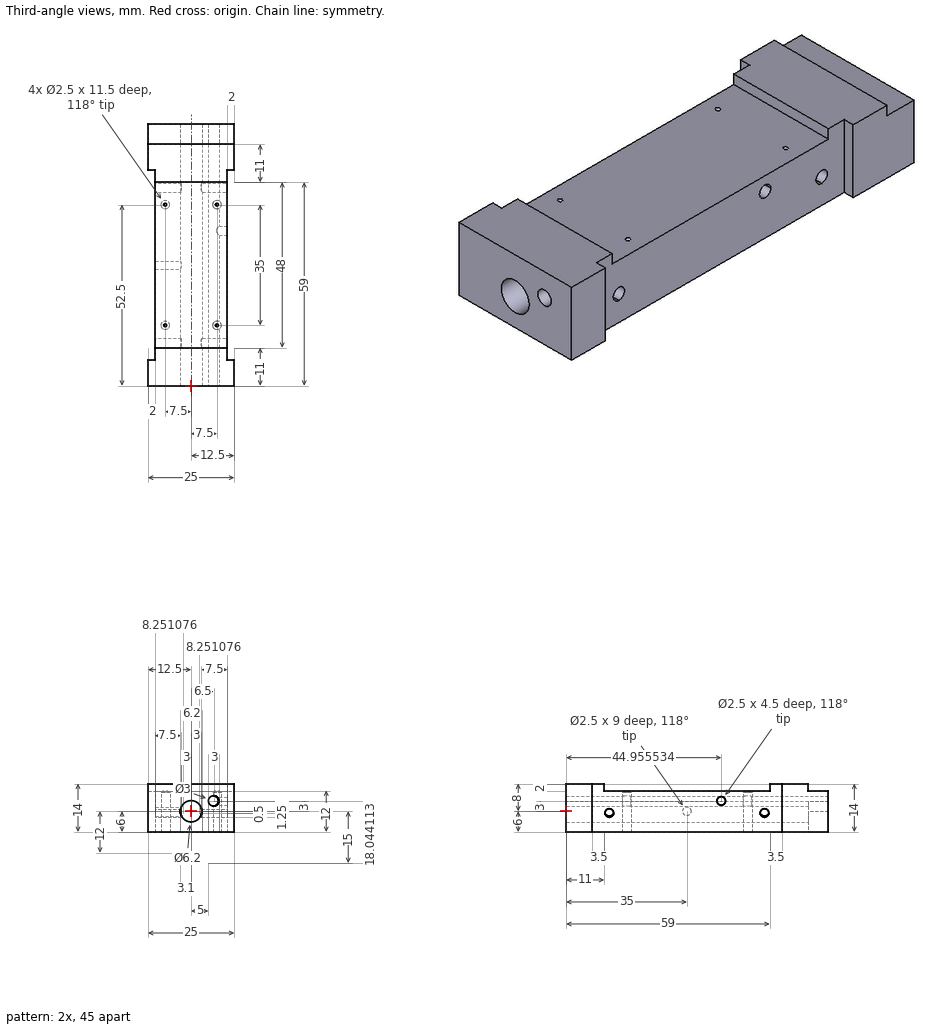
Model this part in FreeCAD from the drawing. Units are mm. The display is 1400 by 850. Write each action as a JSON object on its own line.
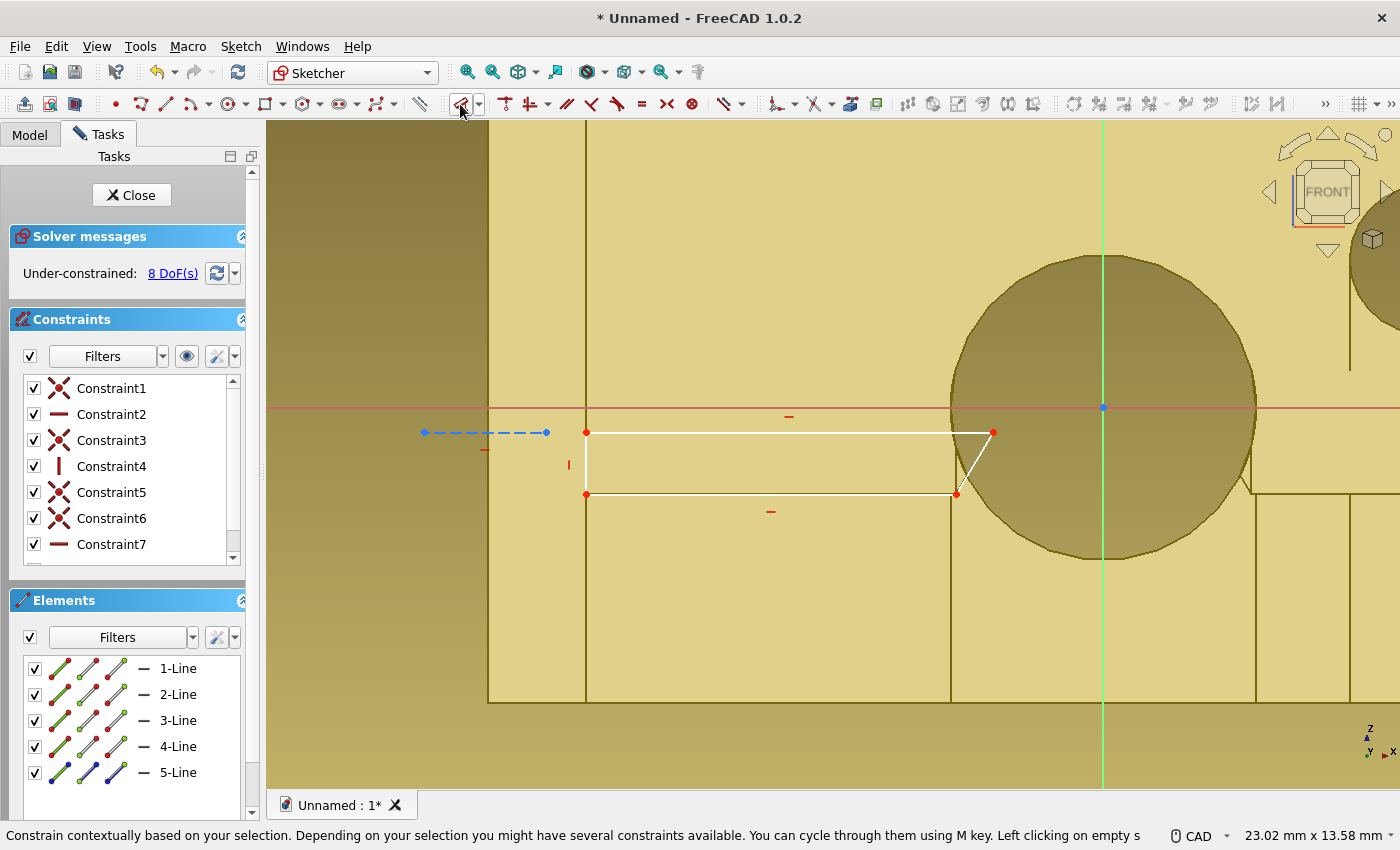
{"action": "left_click", "coordinate": [956, 495]}
{"action": "left_click", "coordinate": [1030, 529]}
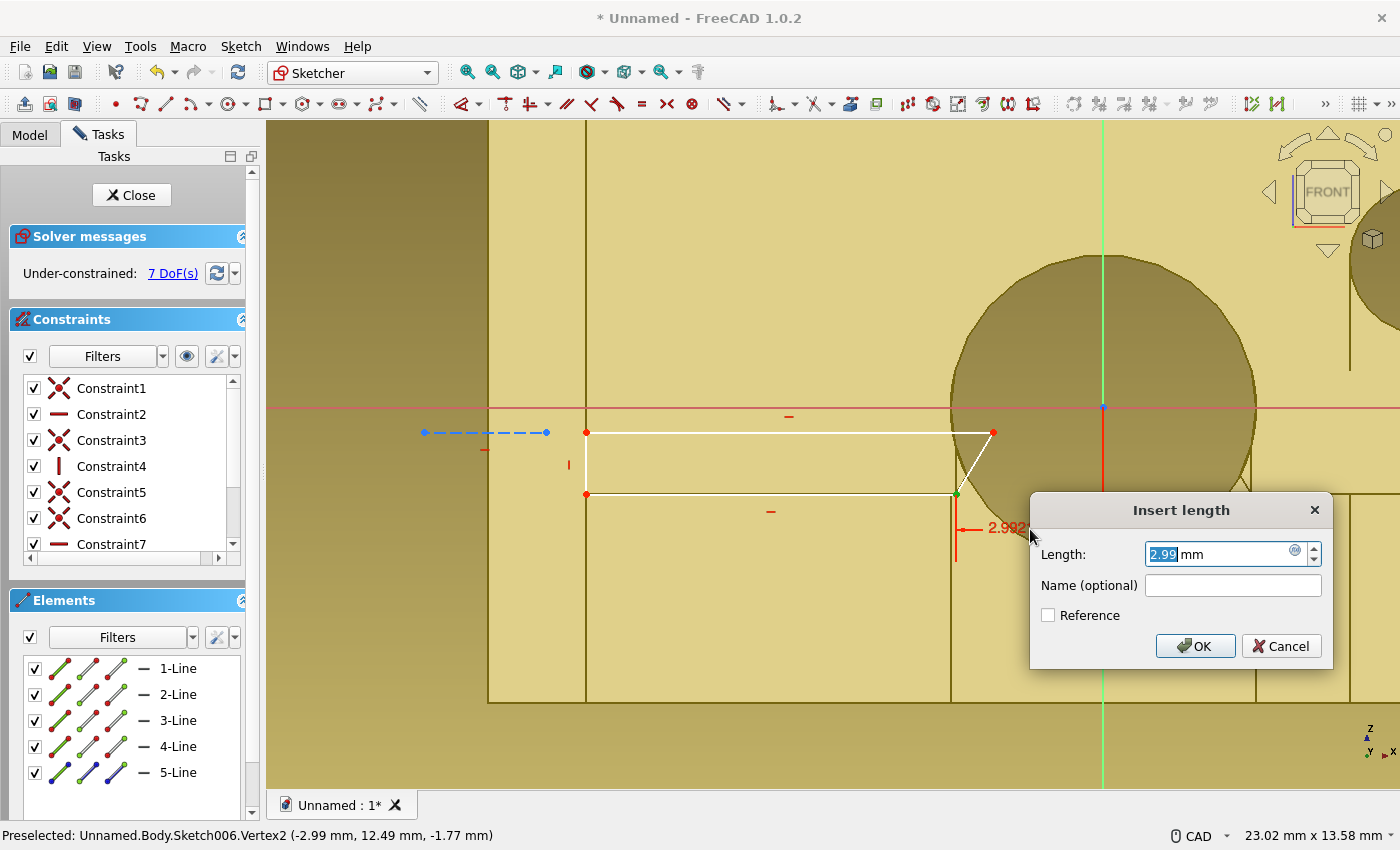
{"action": "type", "text": "3"}
{"action": "key", "text": "Return"}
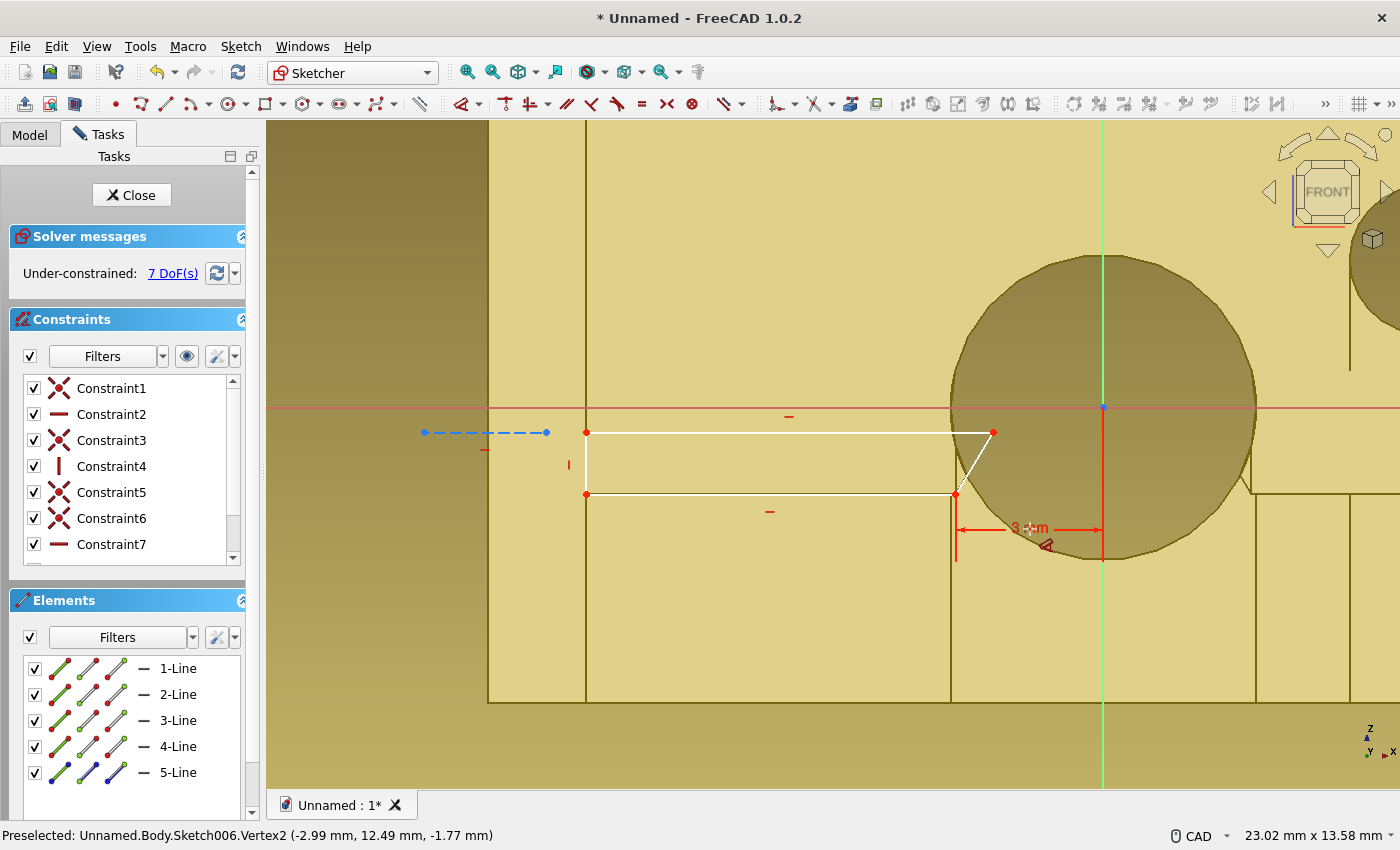
{"action": "left_click", "coordinate": [845, 495]}
{"action": "left_click", "coordinate": [771, 529]}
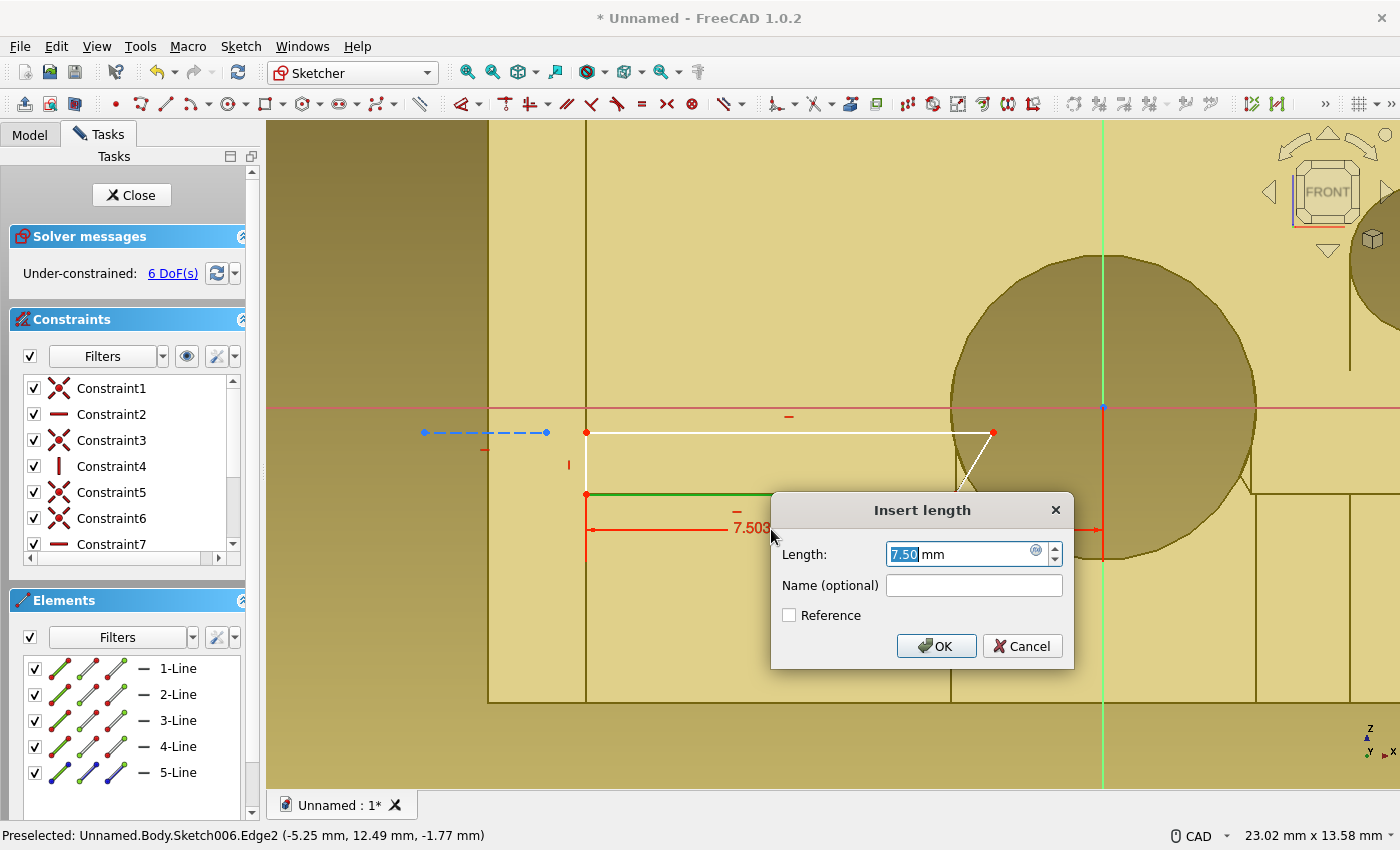
{"action": "type", "text": "7.5"}
{"action": "key", "text": "Return"}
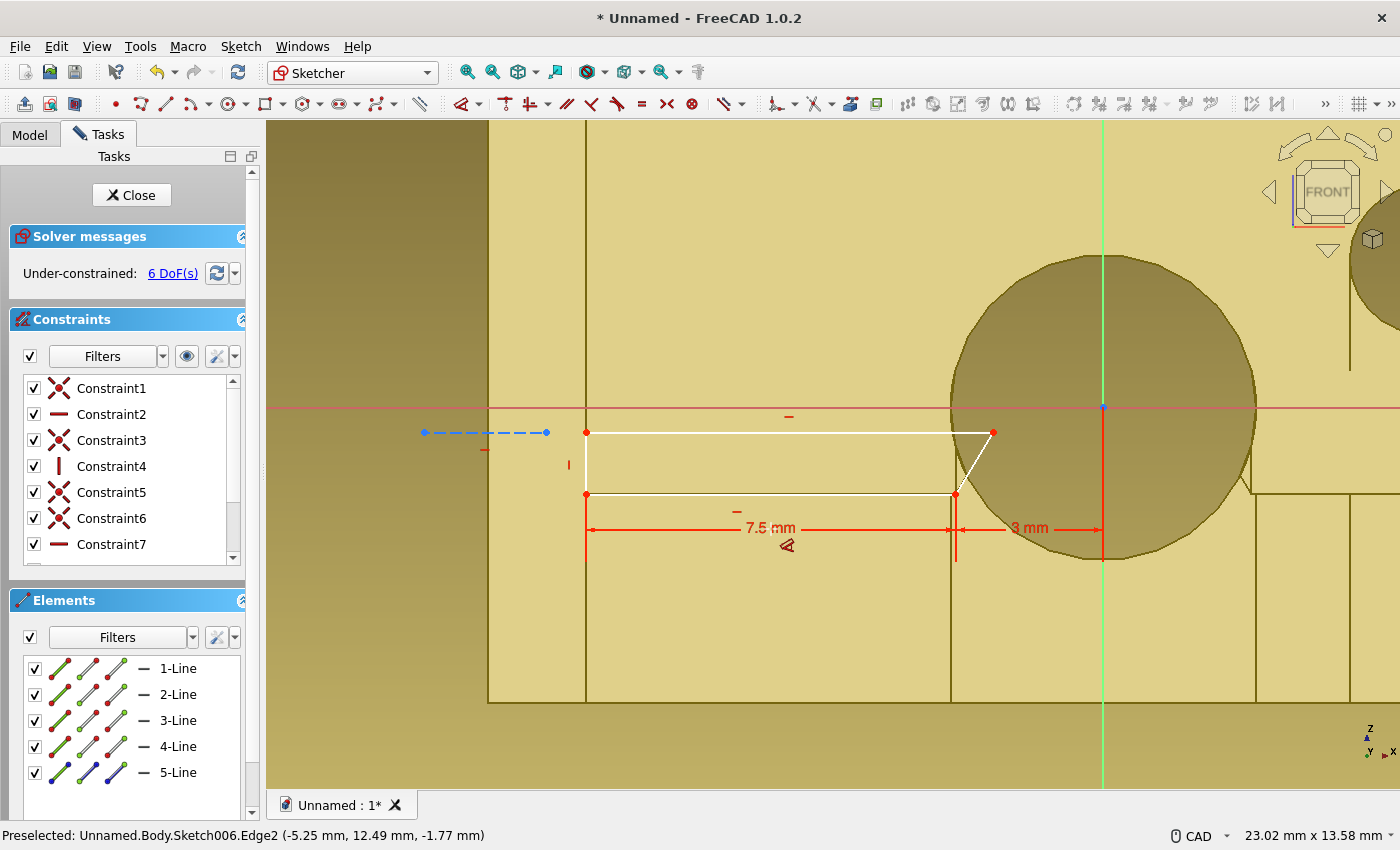
{"action": "left_click", "coordinate": [586, 476]}
{"action": "left_click", "coordinate": [552, 464]}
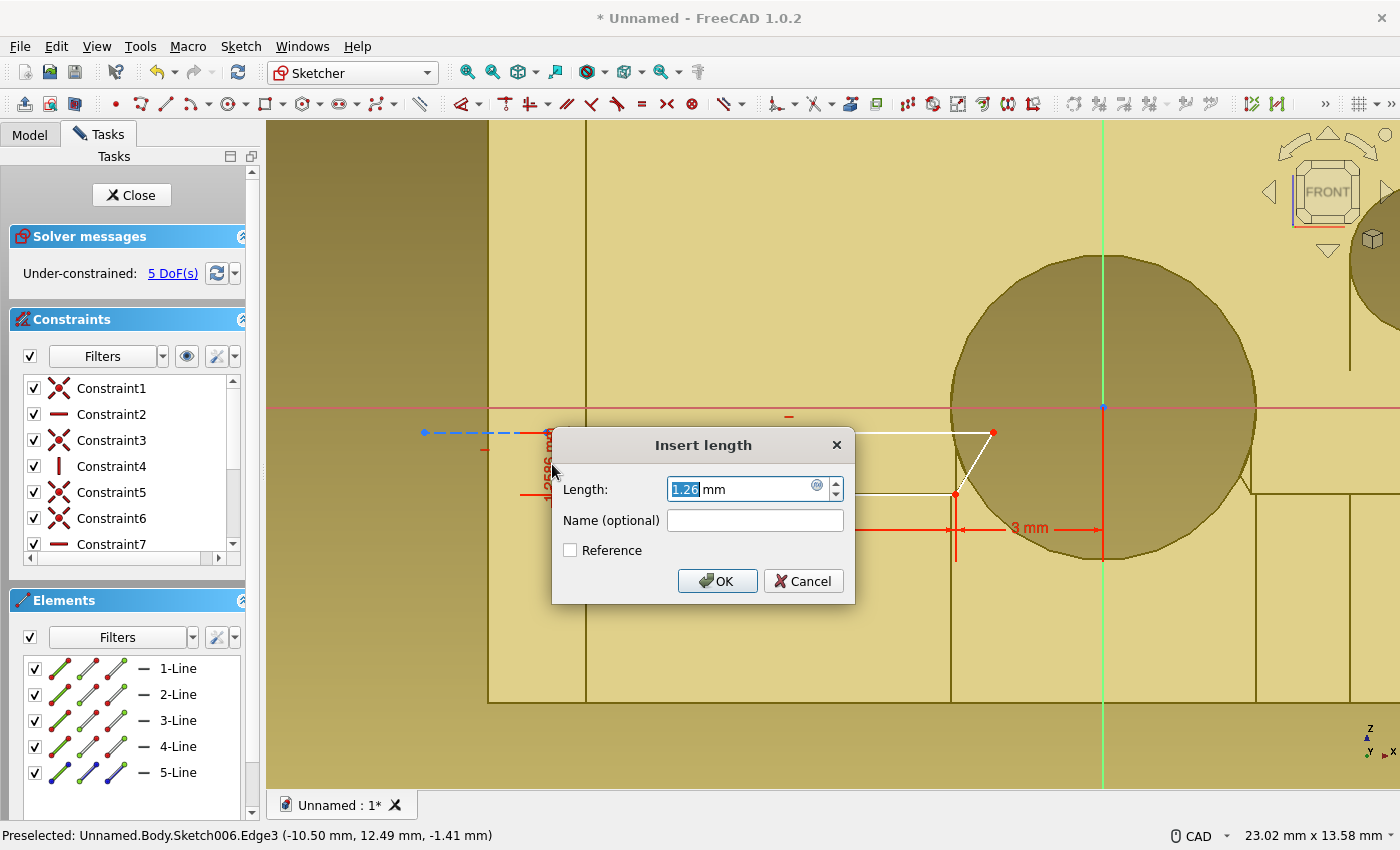
{"action": "type", "text": "1.25"}
{"action": "key", "text": "Return"}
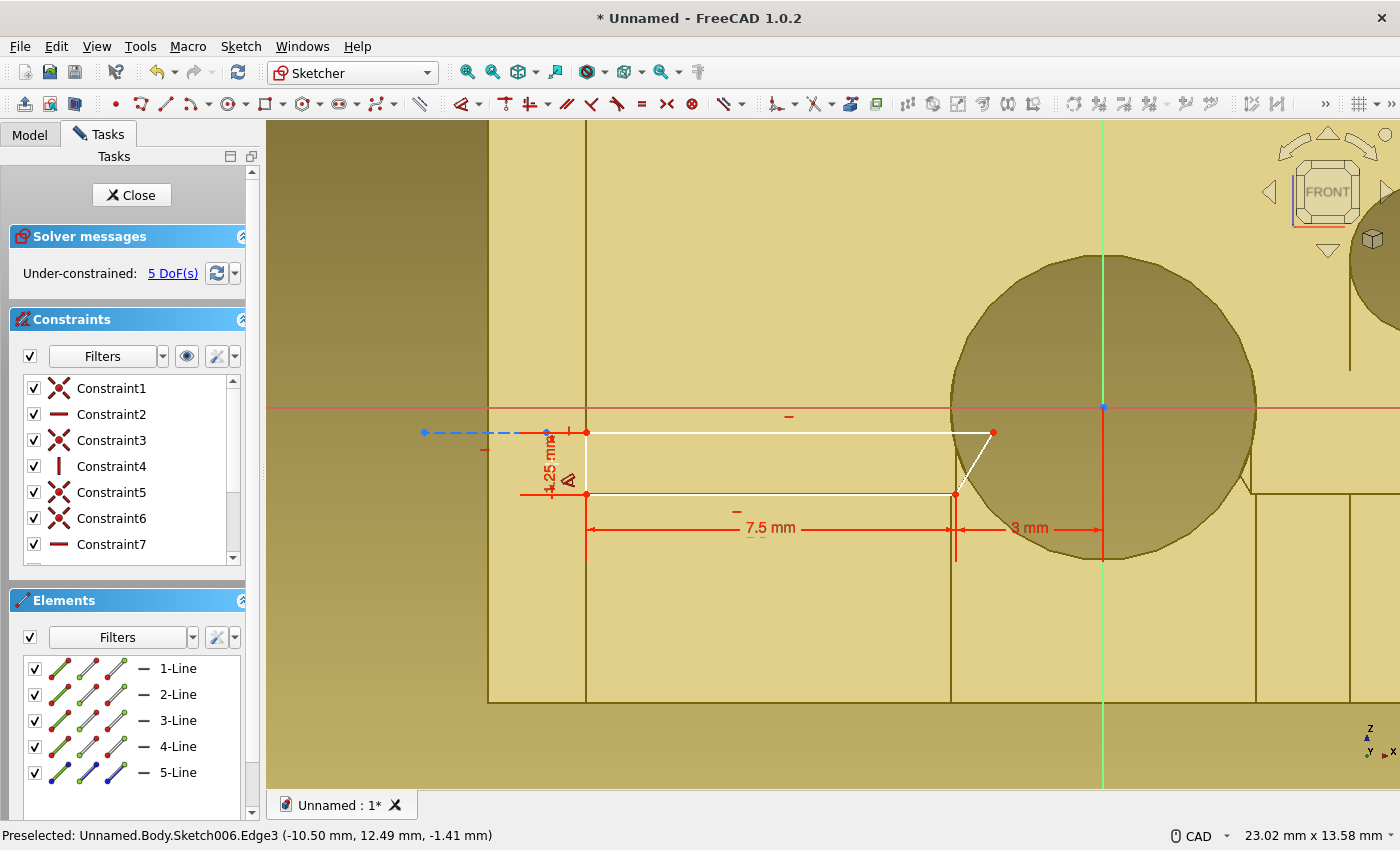
{"action": "scroll", "coordinate": [993, 433], "scroll_direction": "up", "scroll_amount": 3}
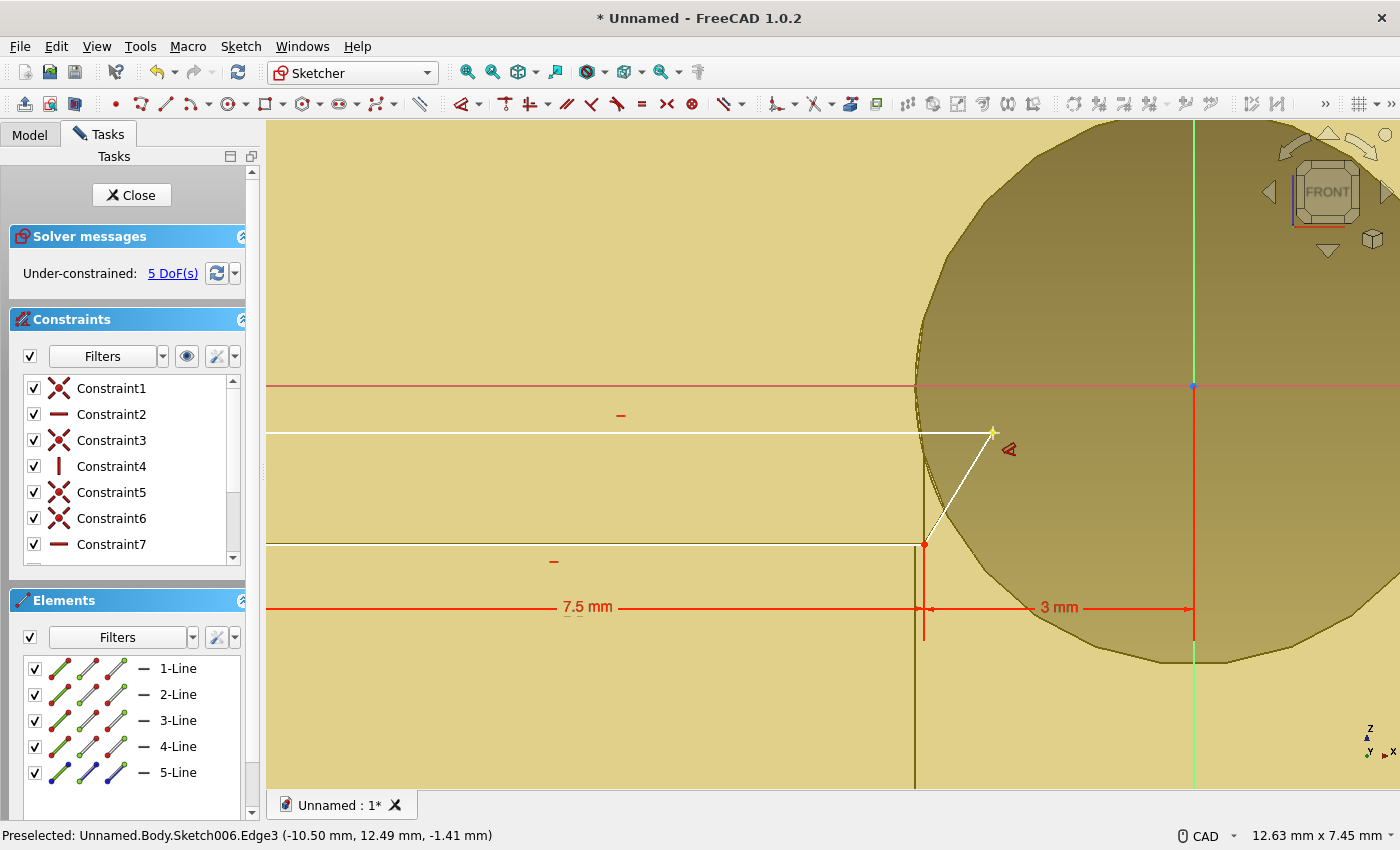
{"action": "left_click", "coordinate": [992, 433]}
{"action": "left_click", "coordinate": [1228, 410]}